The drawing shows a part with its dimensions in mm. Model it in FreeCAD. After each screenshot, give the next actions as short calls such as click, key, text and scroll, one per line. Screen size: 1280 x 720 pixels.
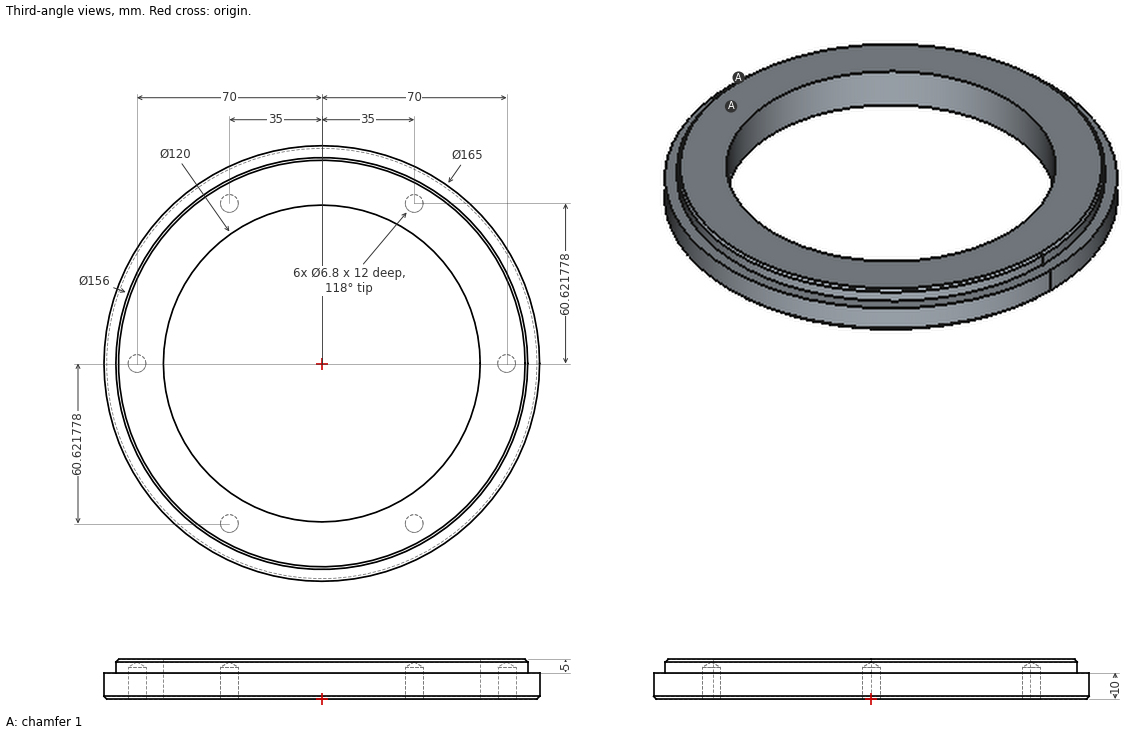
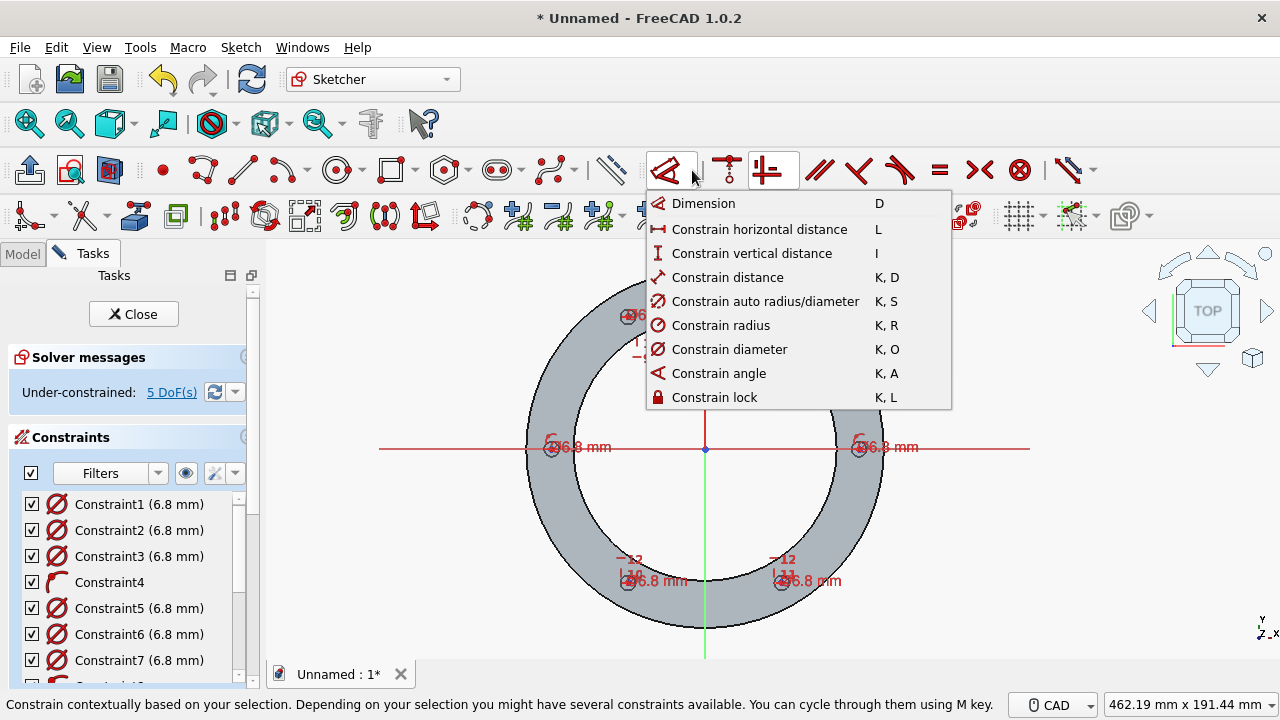
click(799, 229)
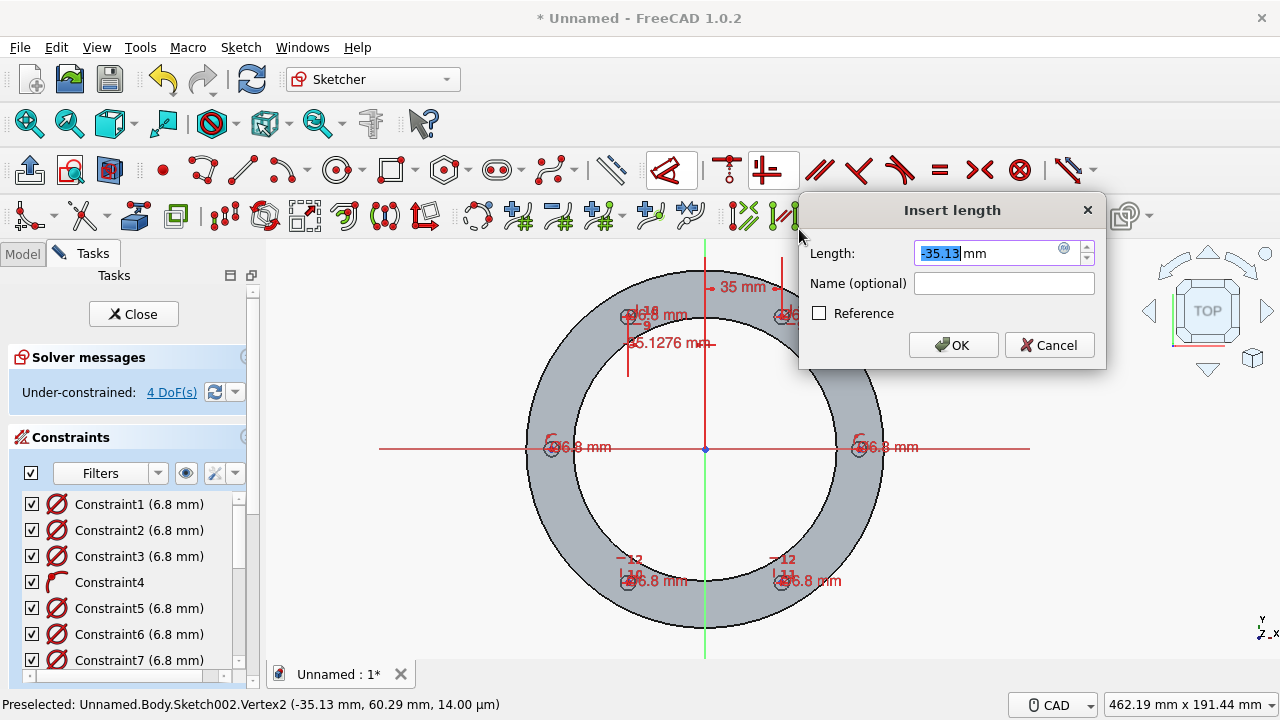
text(-35)
key(Return)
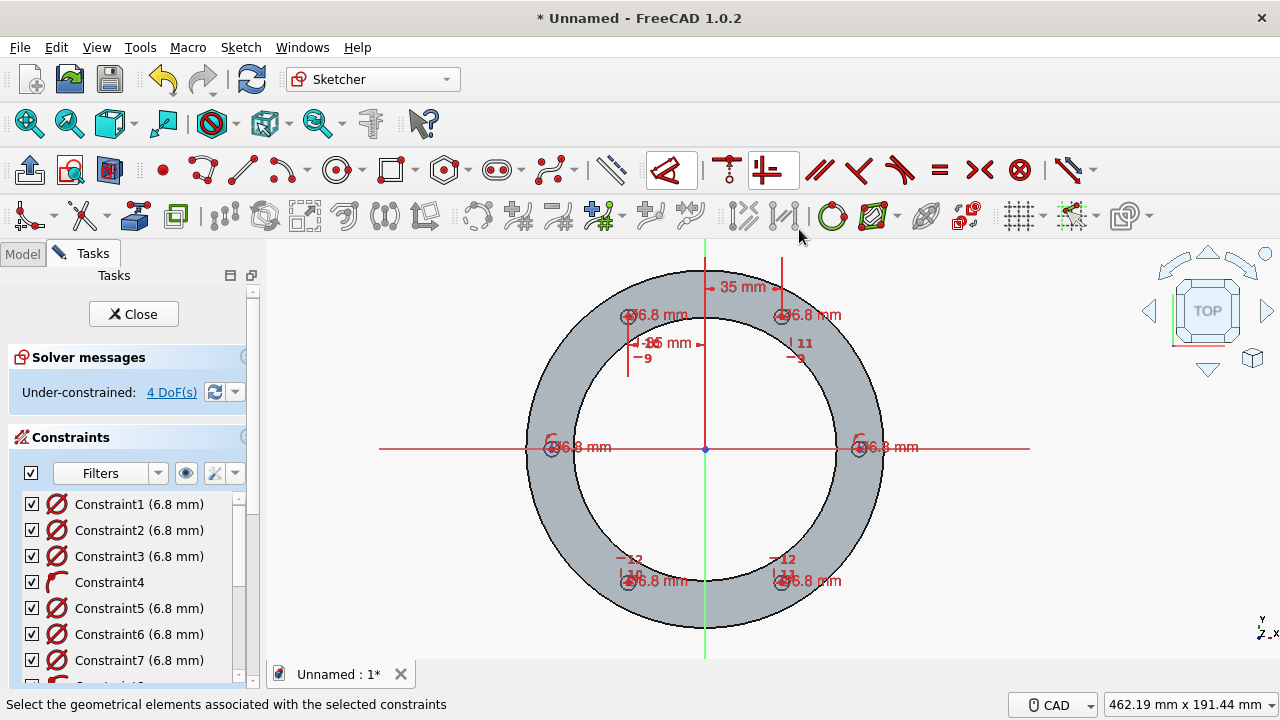
click(552, 449)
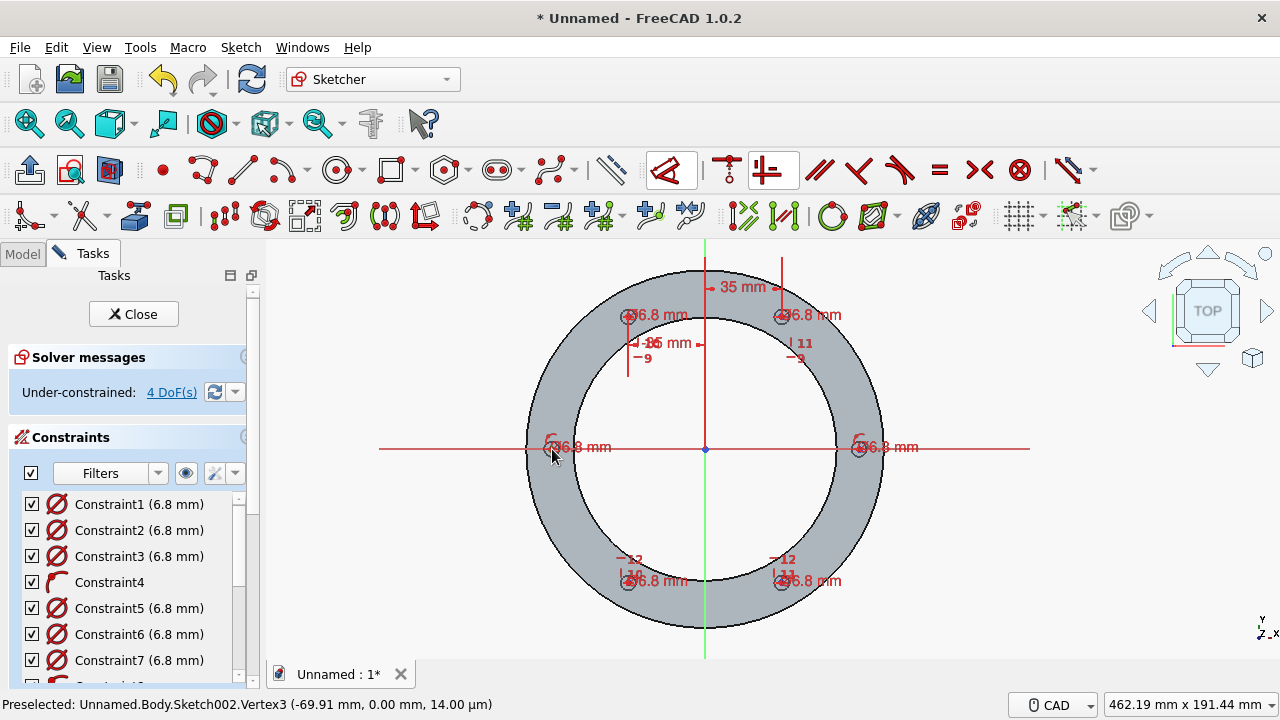
click(692, 170)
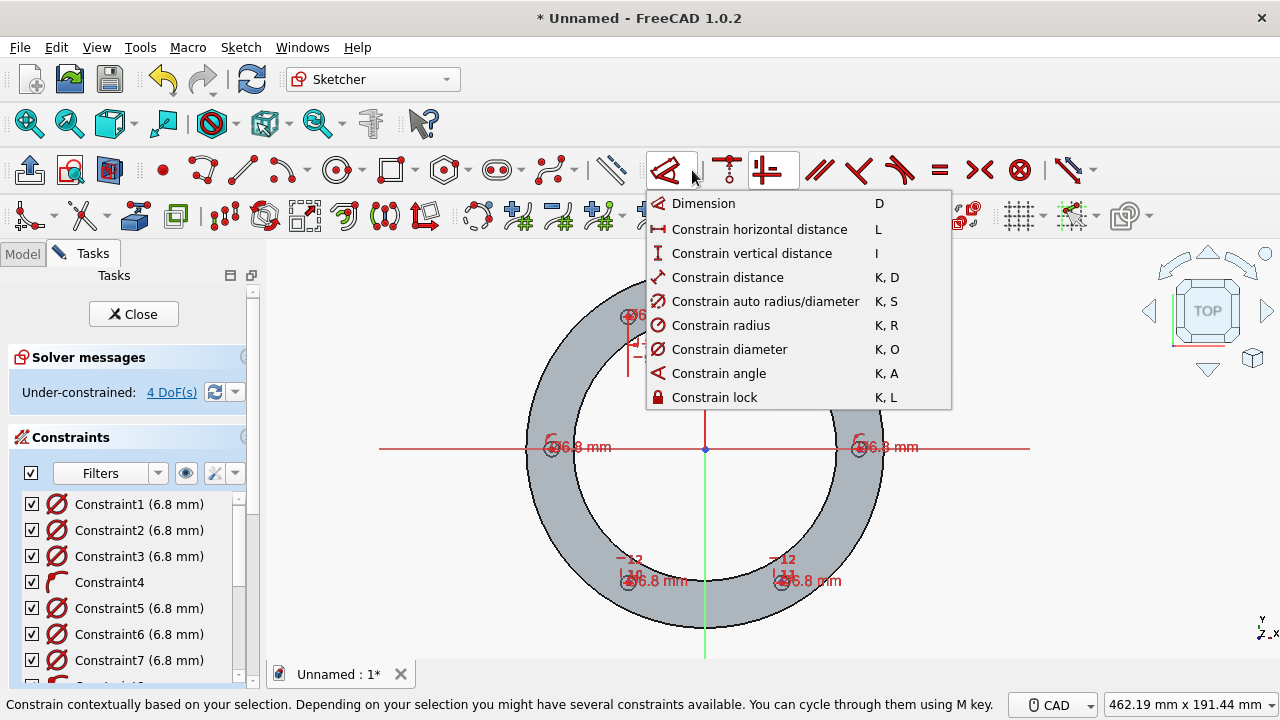
click(799, 229)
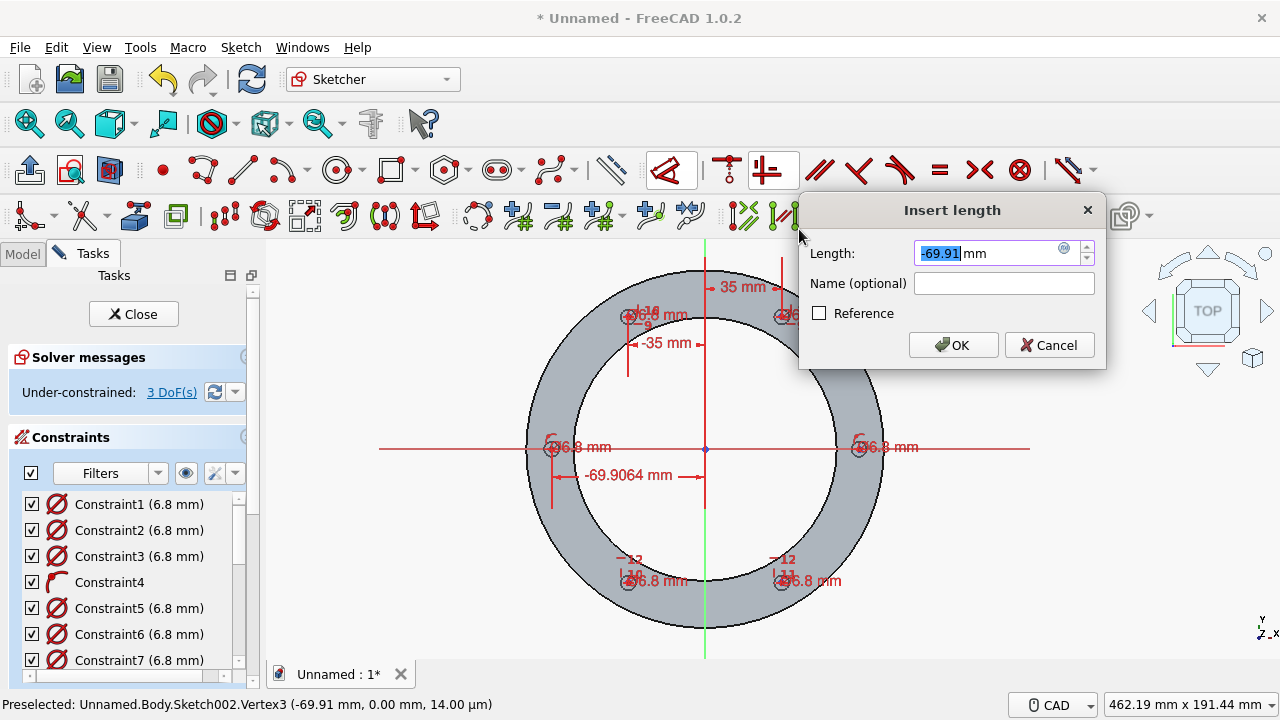
text(-70)
key(Return)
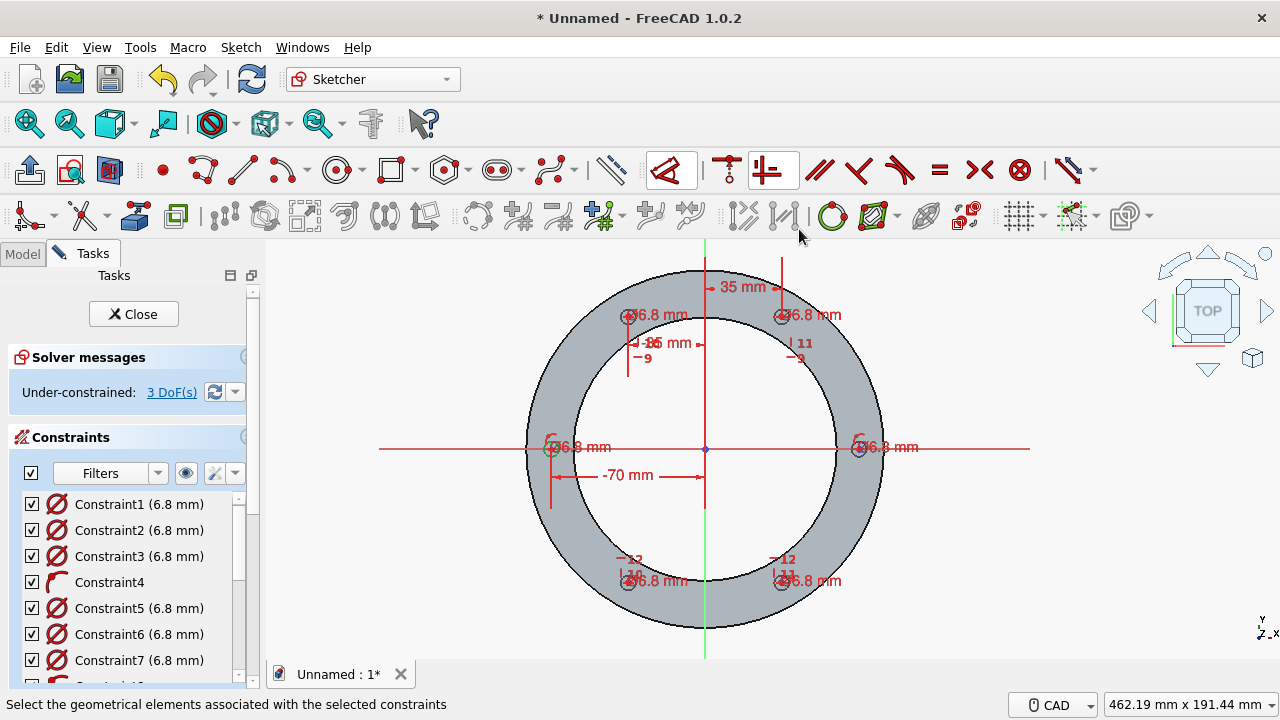
click(859, 449)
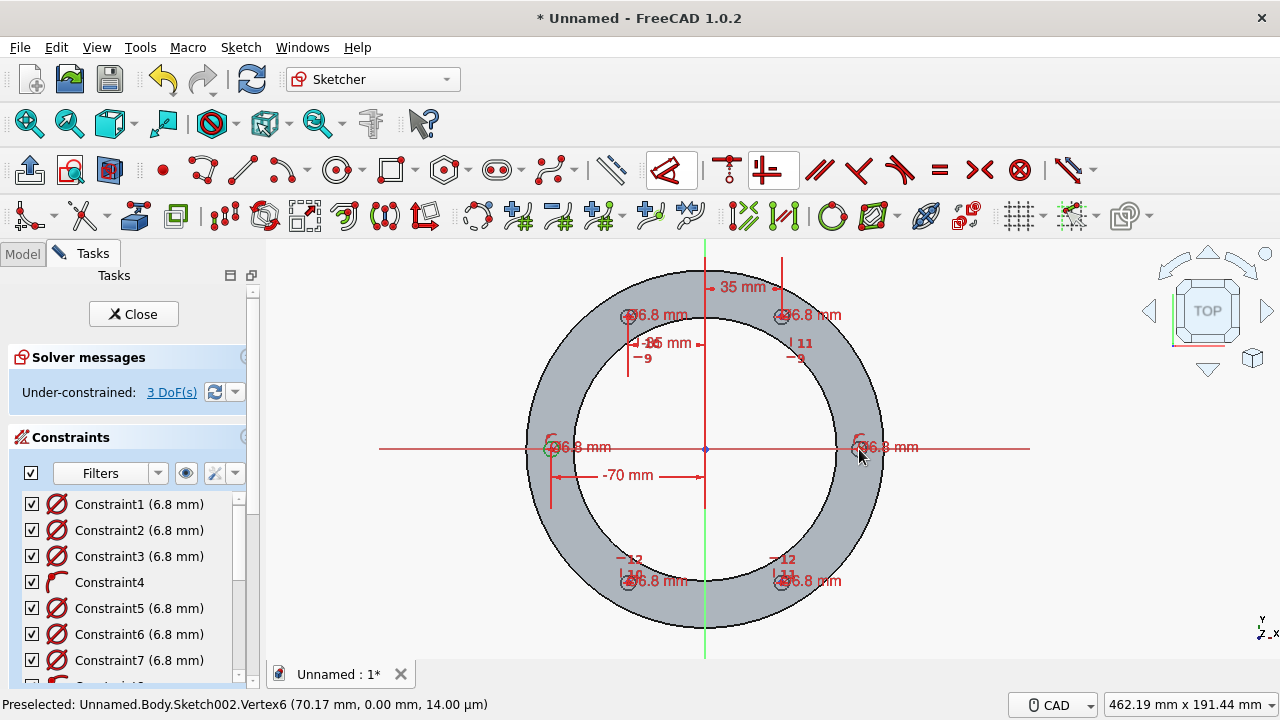
click(692, 170)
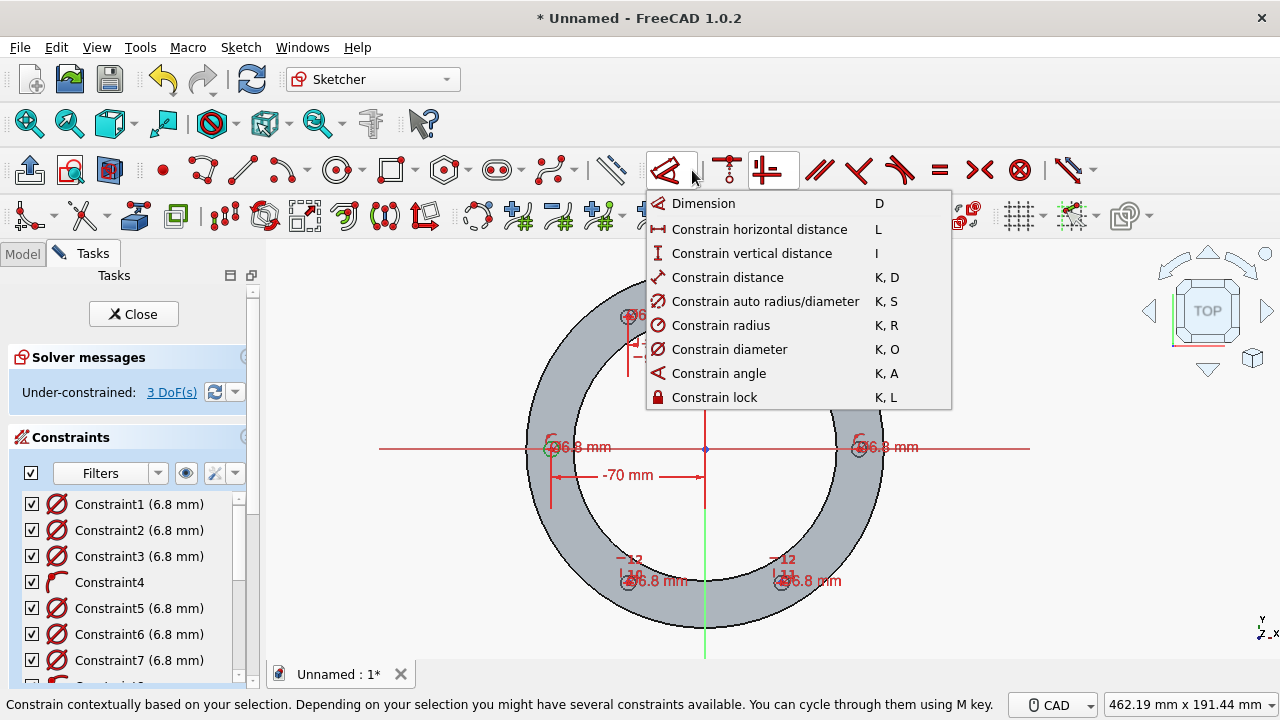
click(799, 229)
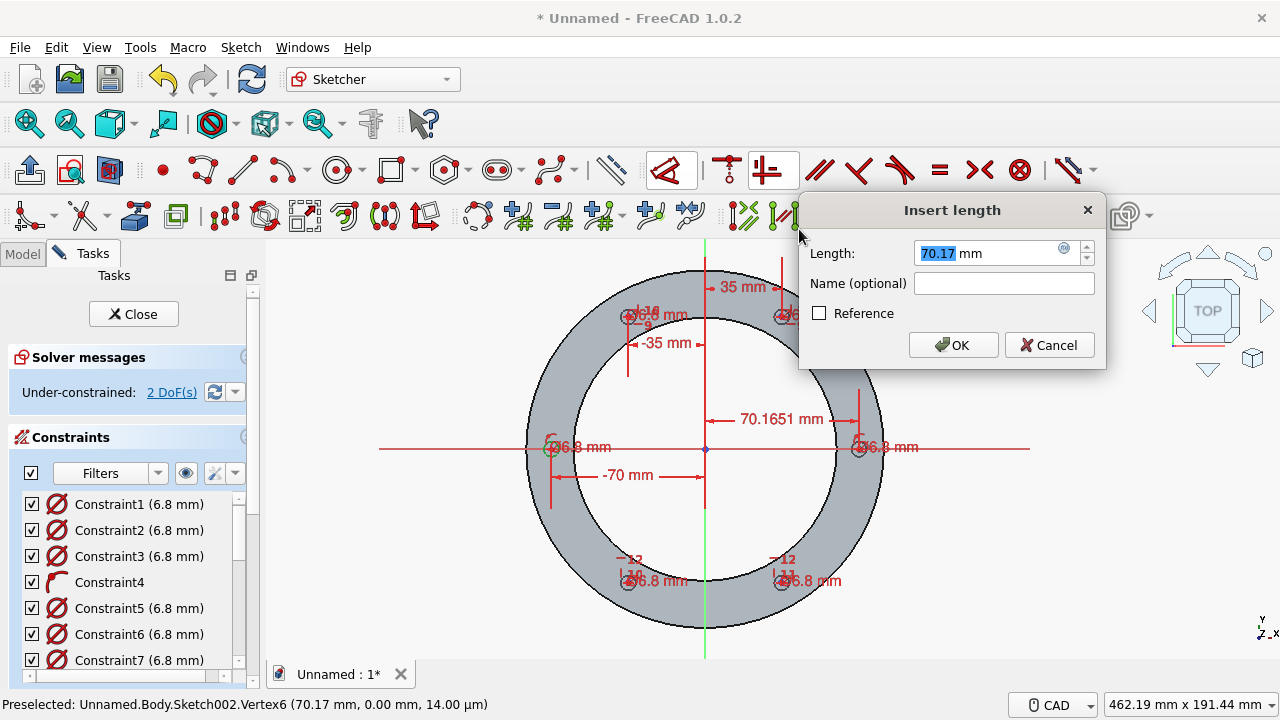
text(70)
key(Return)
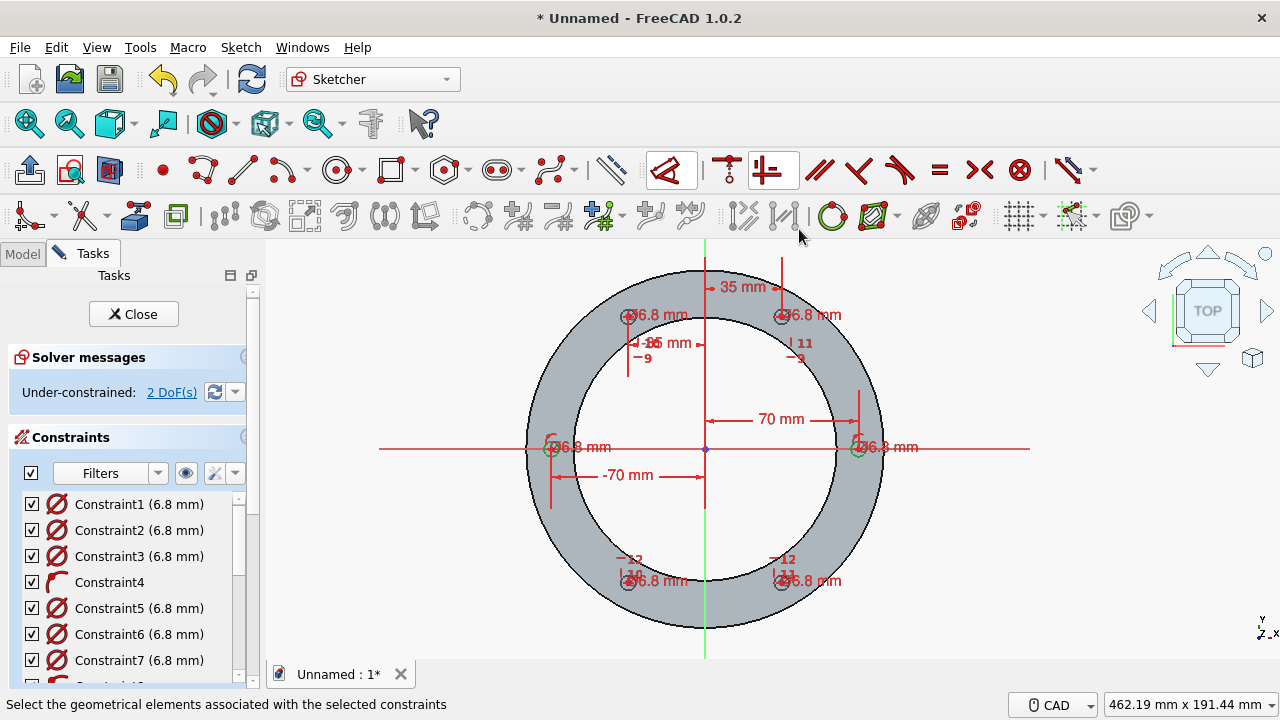
click(782, 317)